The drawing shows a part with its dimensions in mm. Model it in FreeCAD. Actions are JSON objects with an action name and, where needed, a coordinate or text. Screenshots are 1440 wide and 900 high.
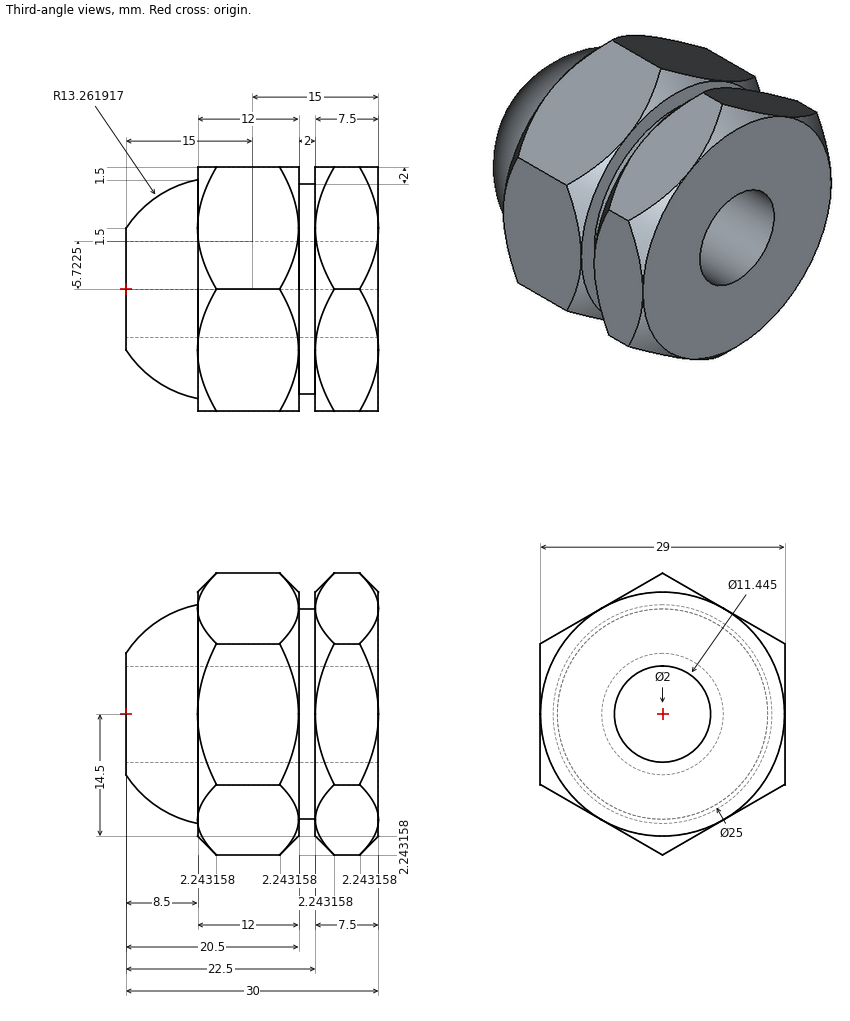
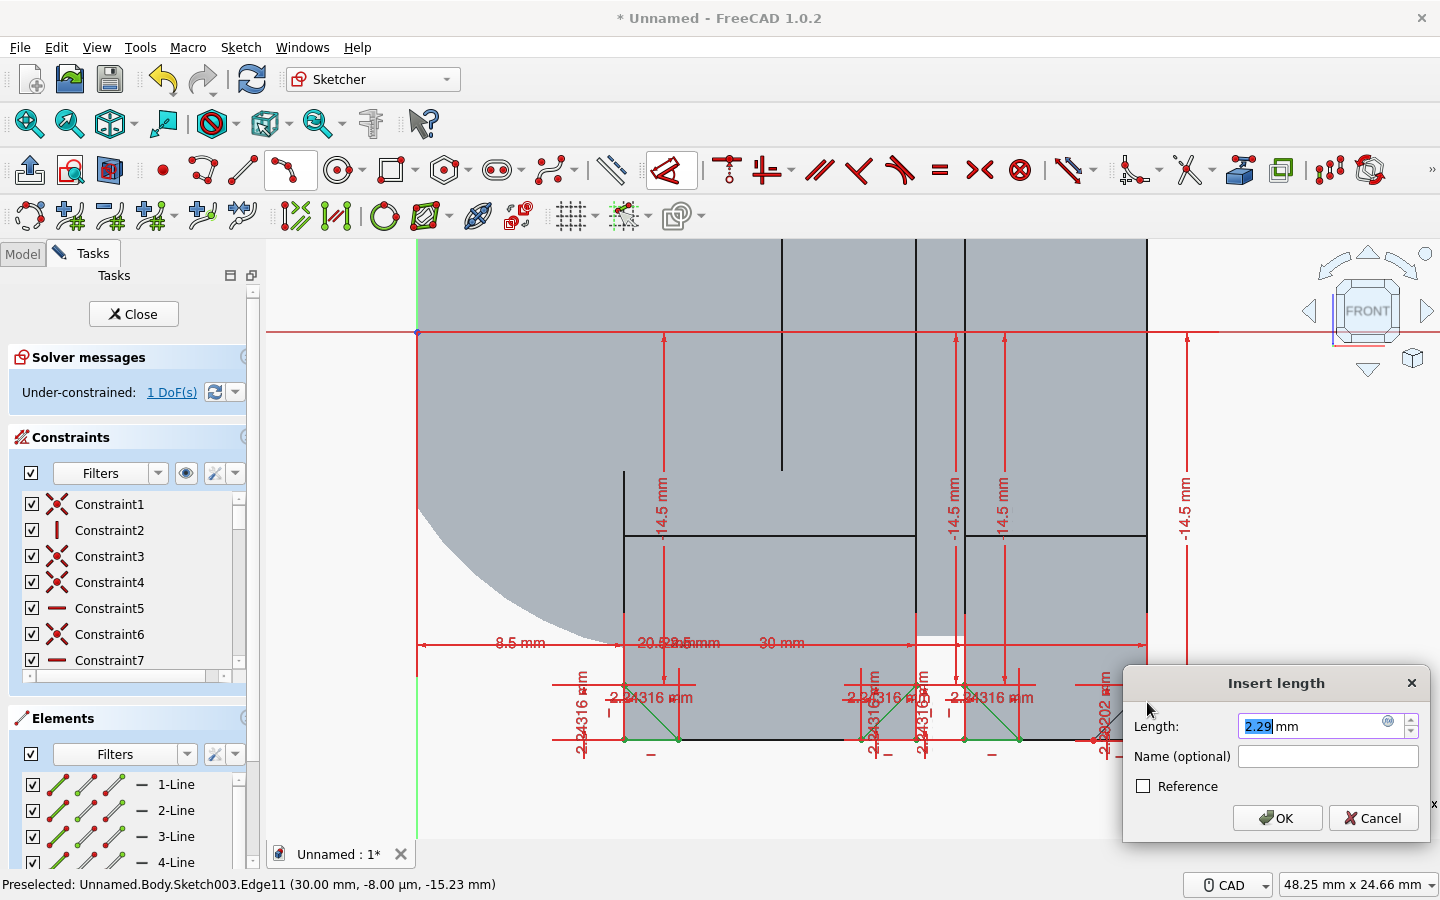
{"action": "type", "text": "2.243158"}
{"action": "key", "text": "Return"}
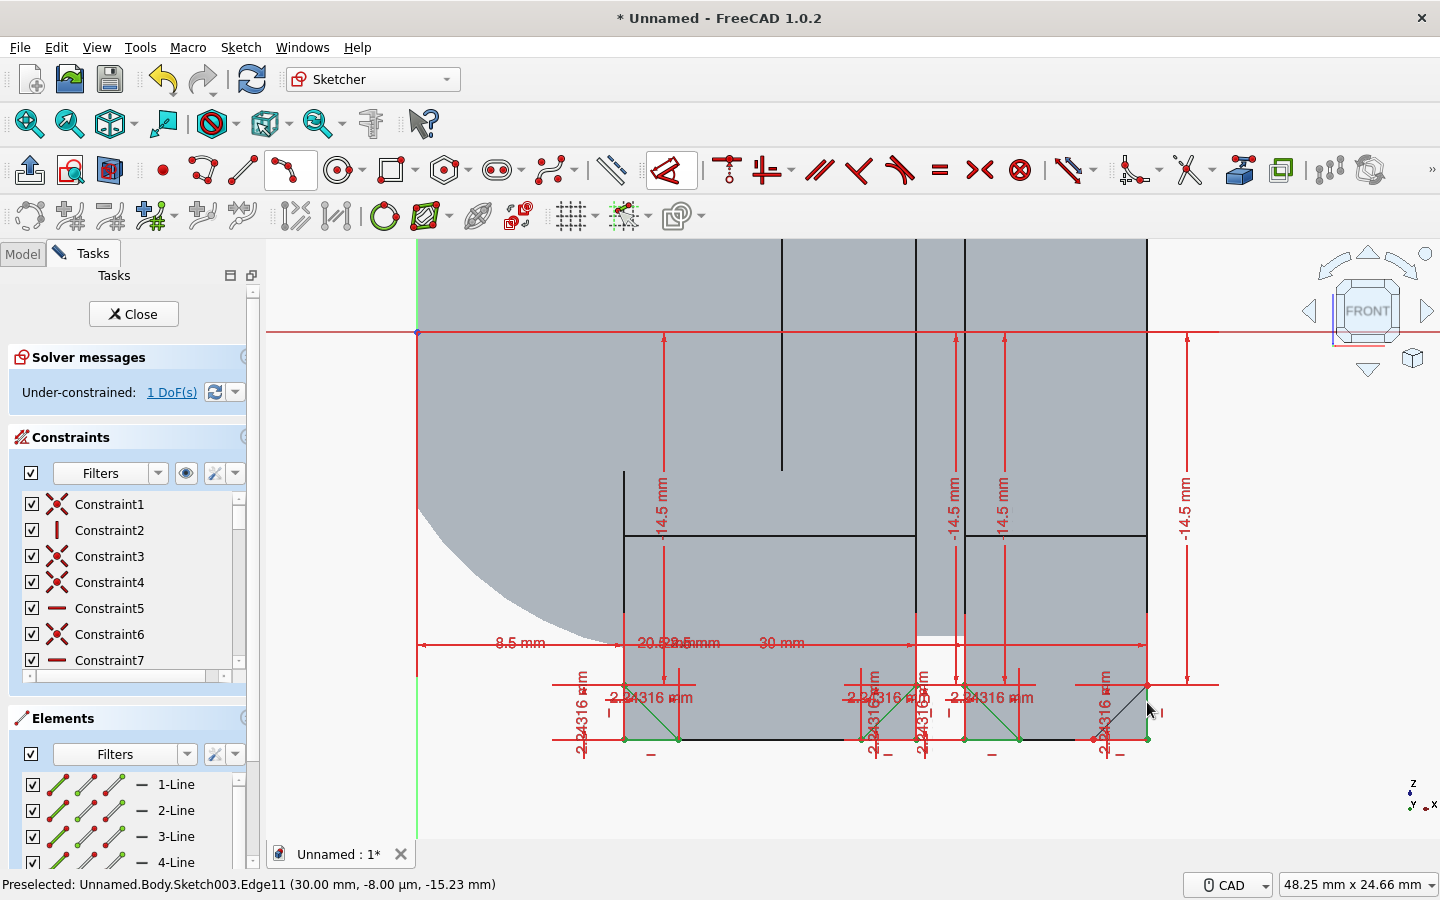
{"action": "left_click", "coordinate": [1131, 740]}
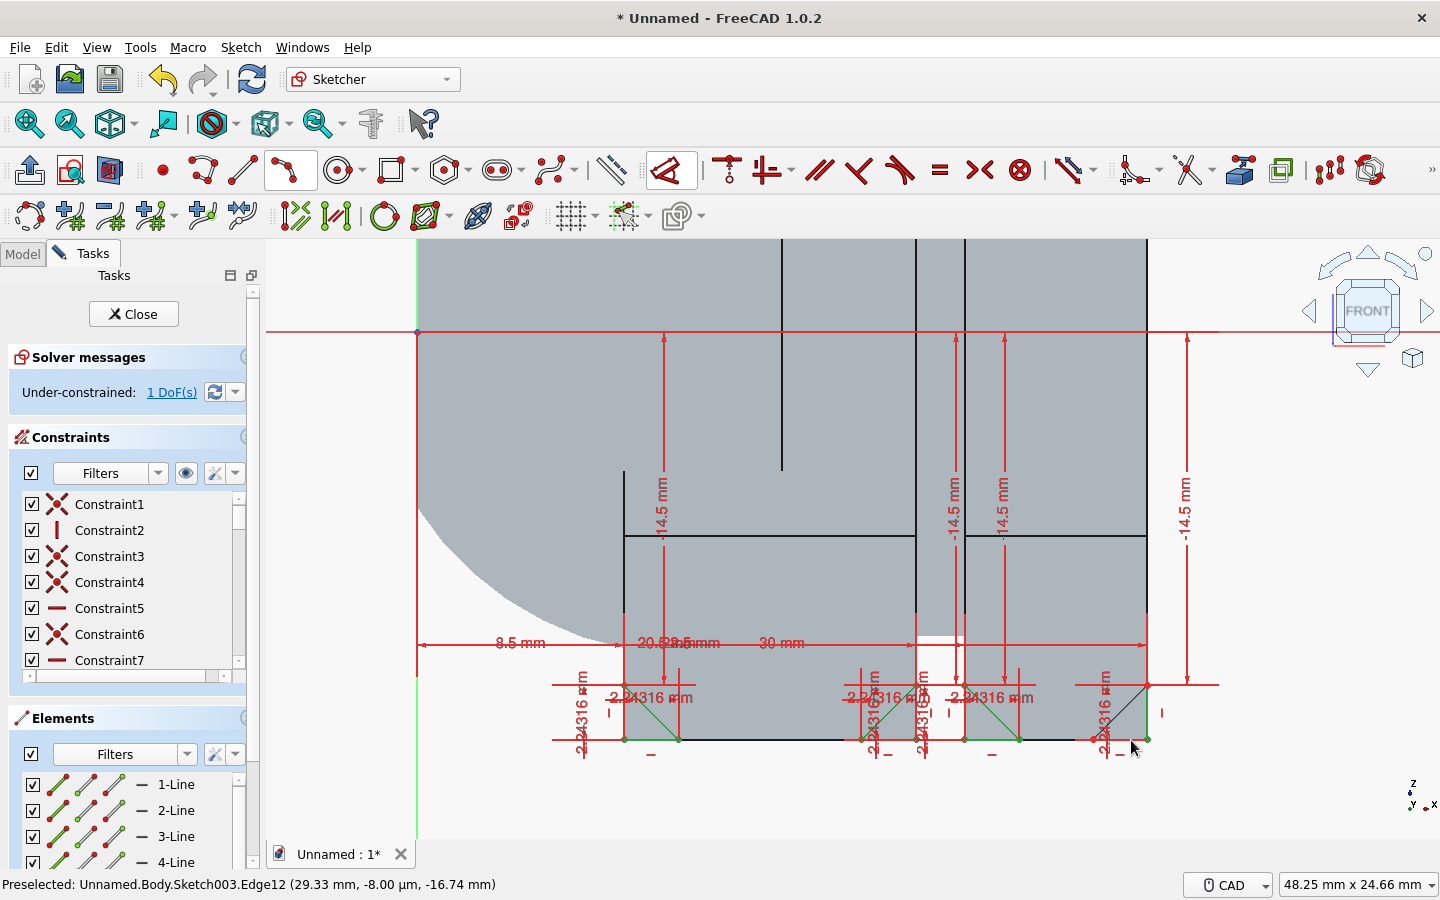
{"action": "key", "text": "l"}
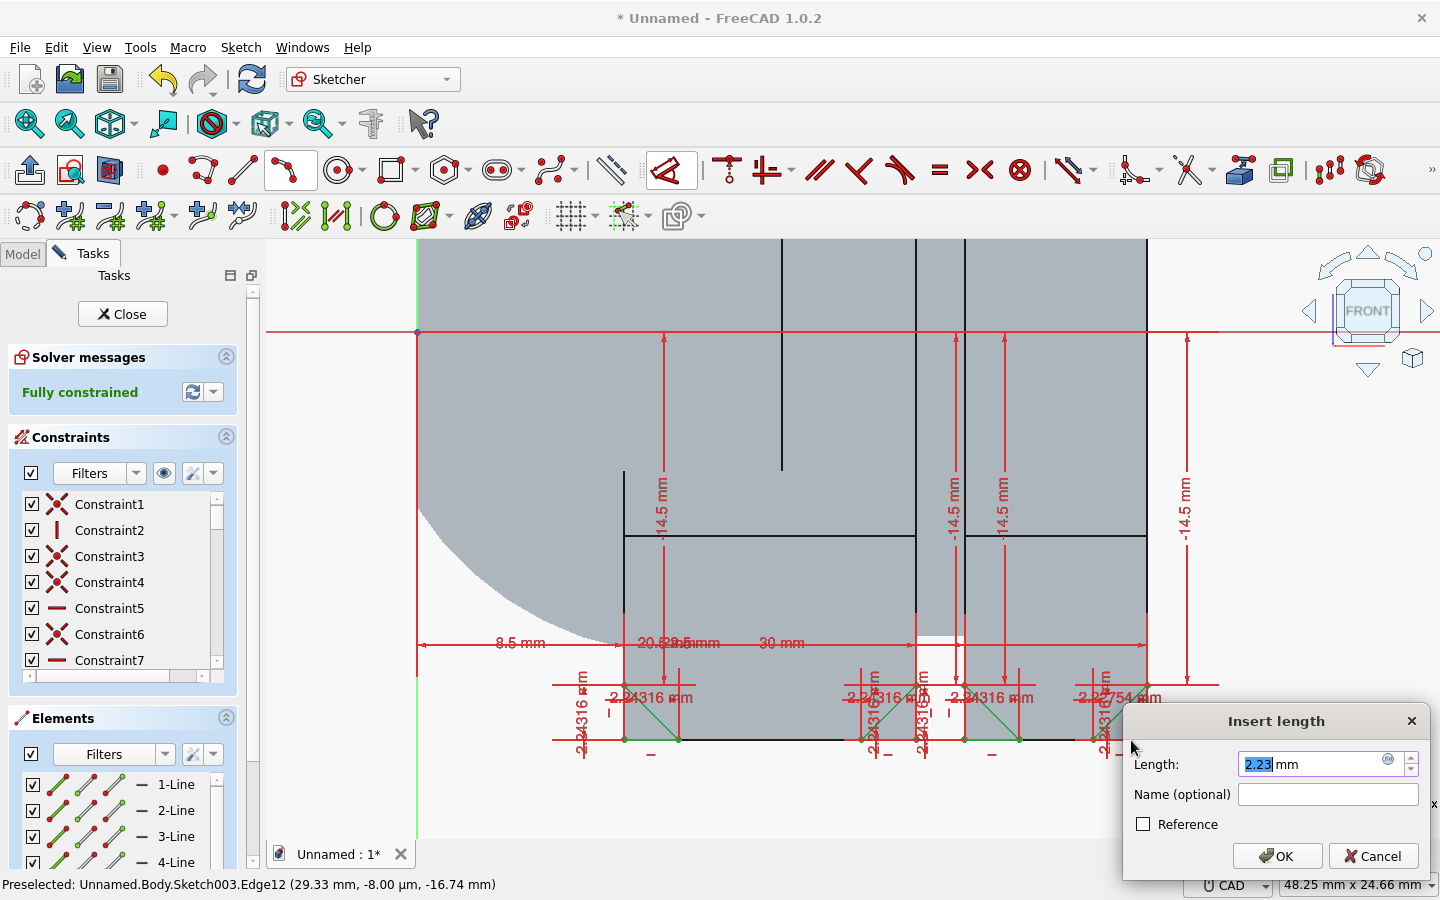
{"action": "type", "text": "2.243158"}
{"action": "key", "text": "Return"}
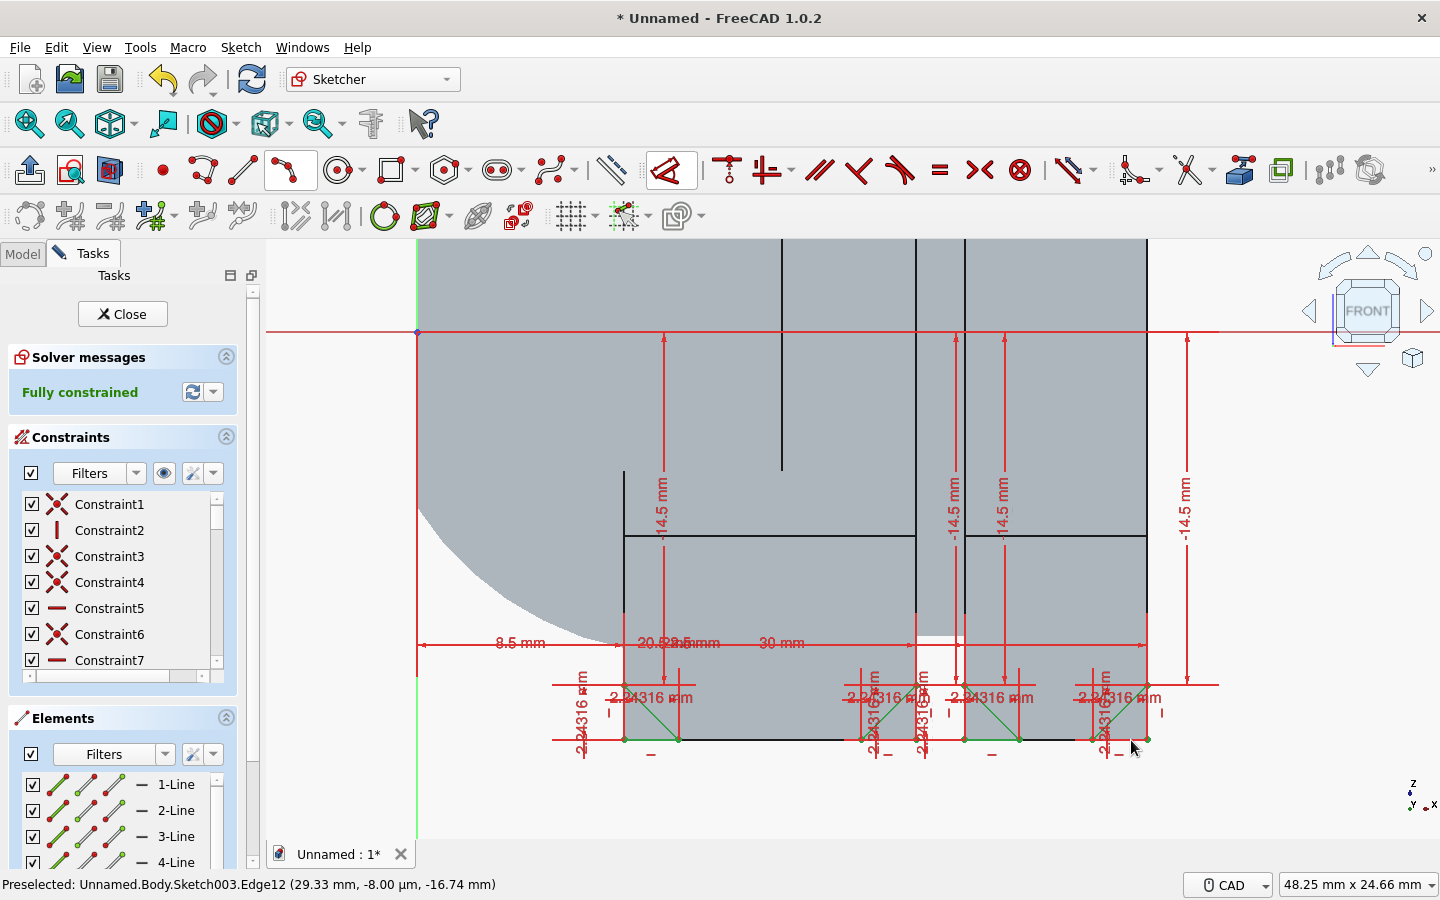
{"action": "left_click", "coordinate": [123, 314]}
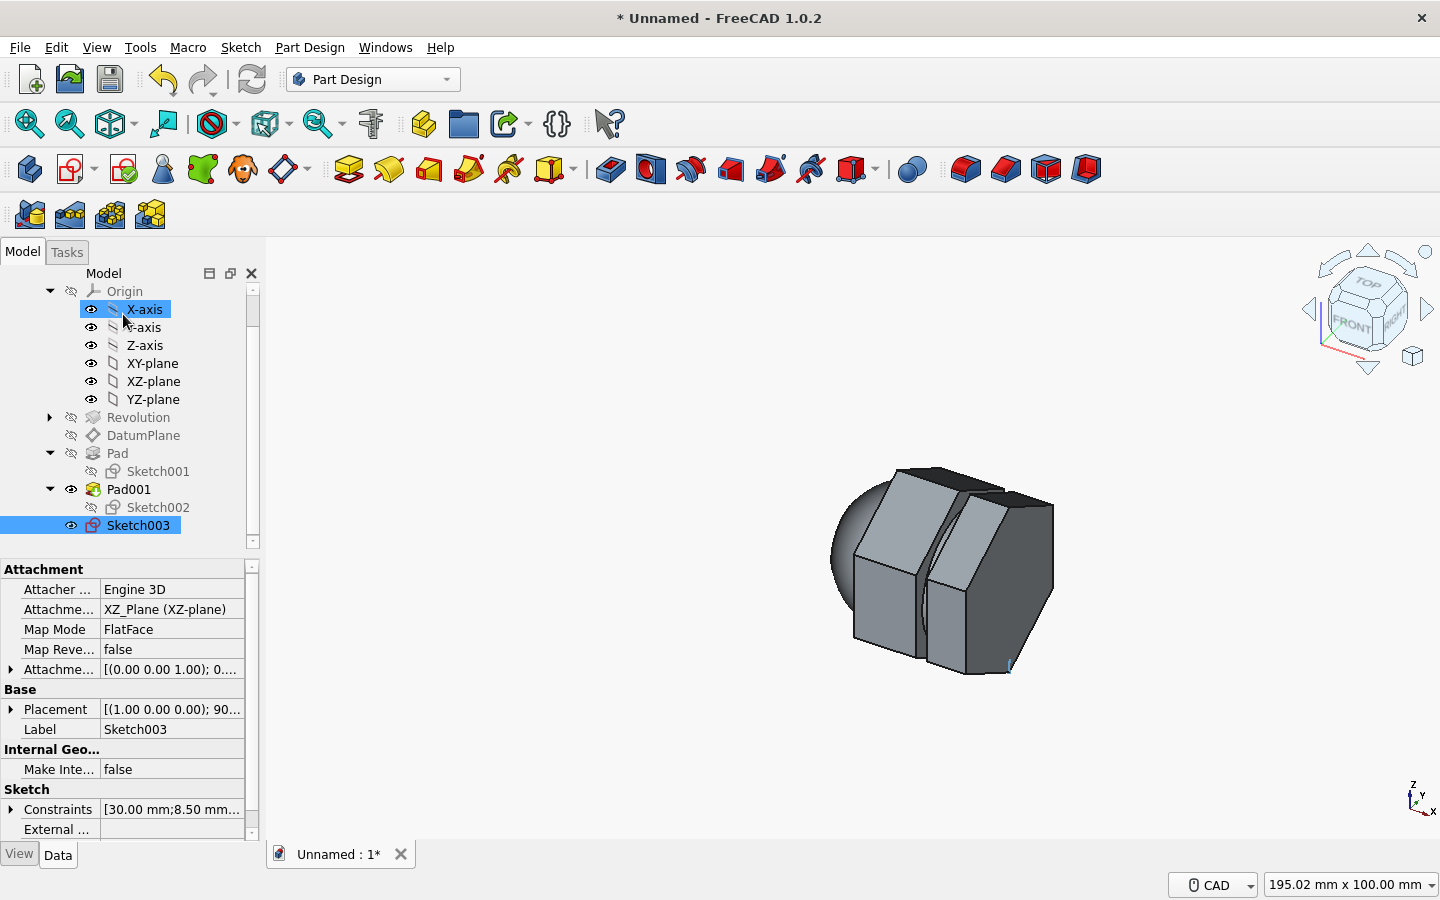
{"action": "left_click", "coordinate": [692, 170]}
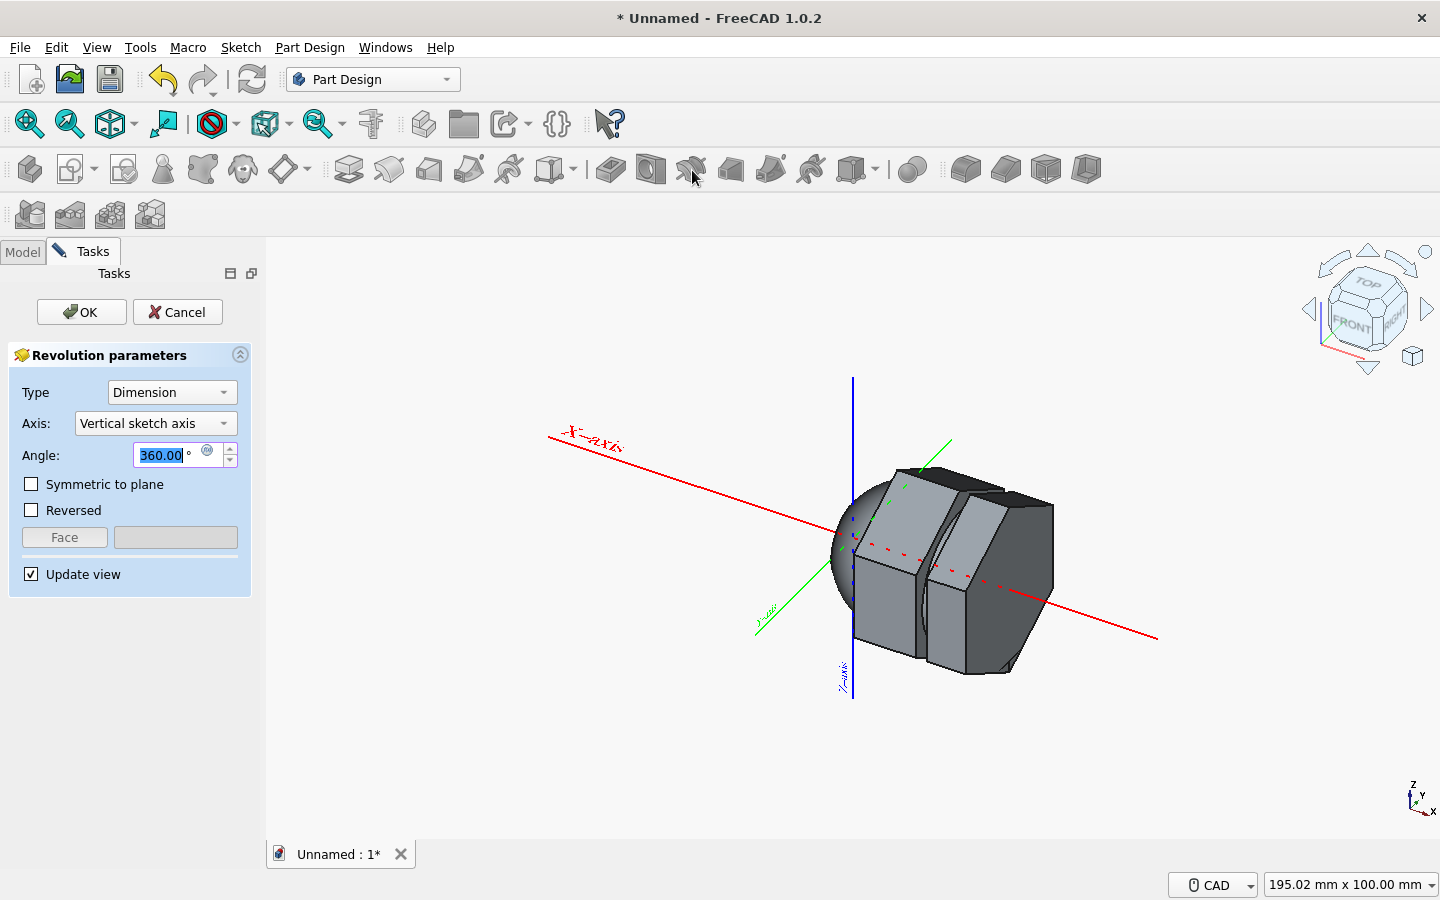
{"action": "left_click", "coordinate": [156, 424]}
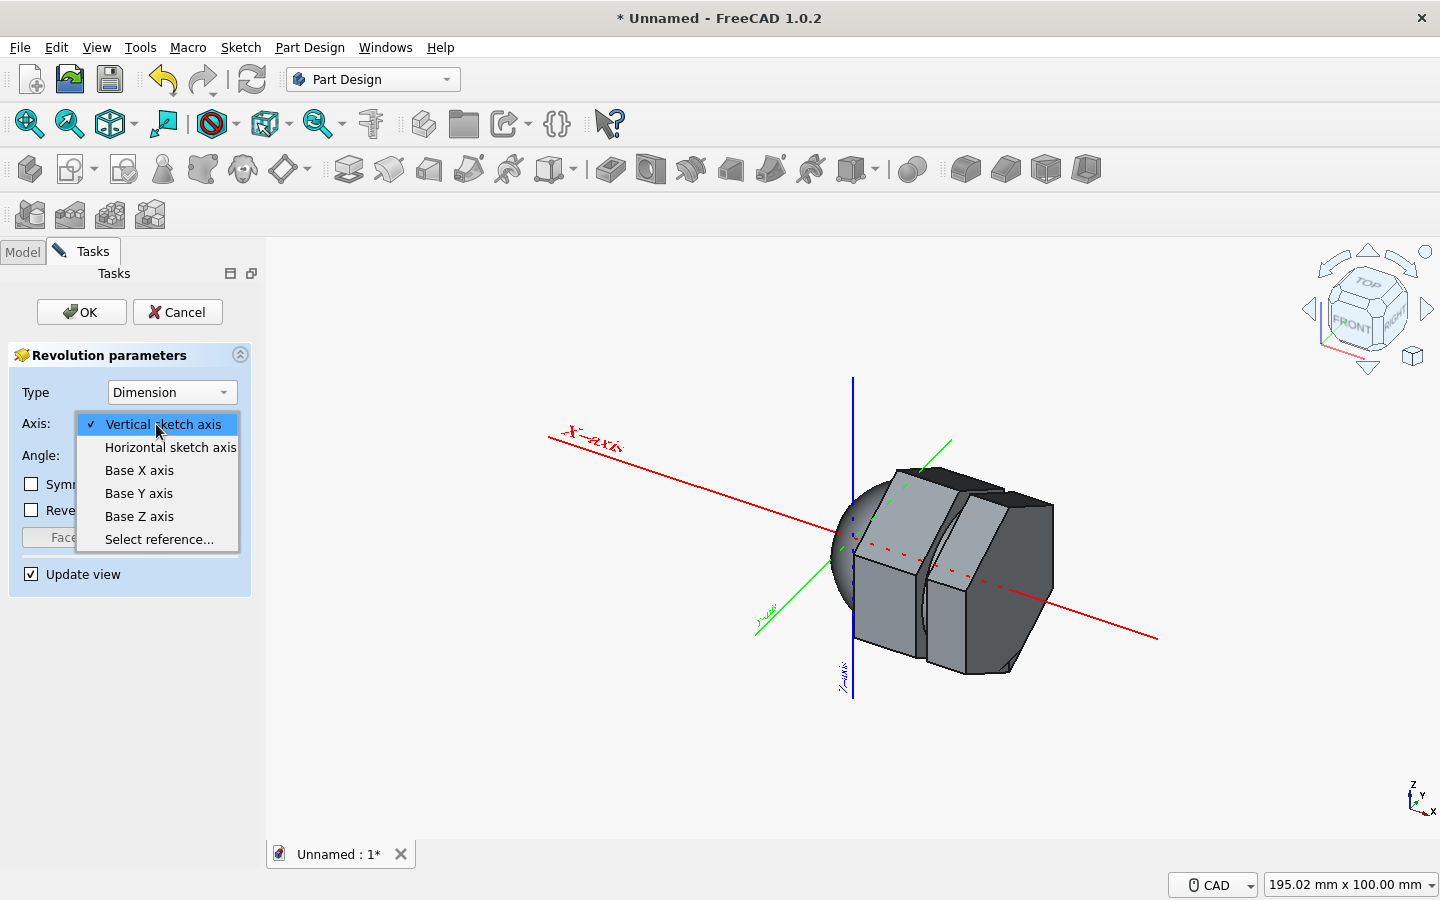
{"action": "left_click", "coordinate": [156, 448]}